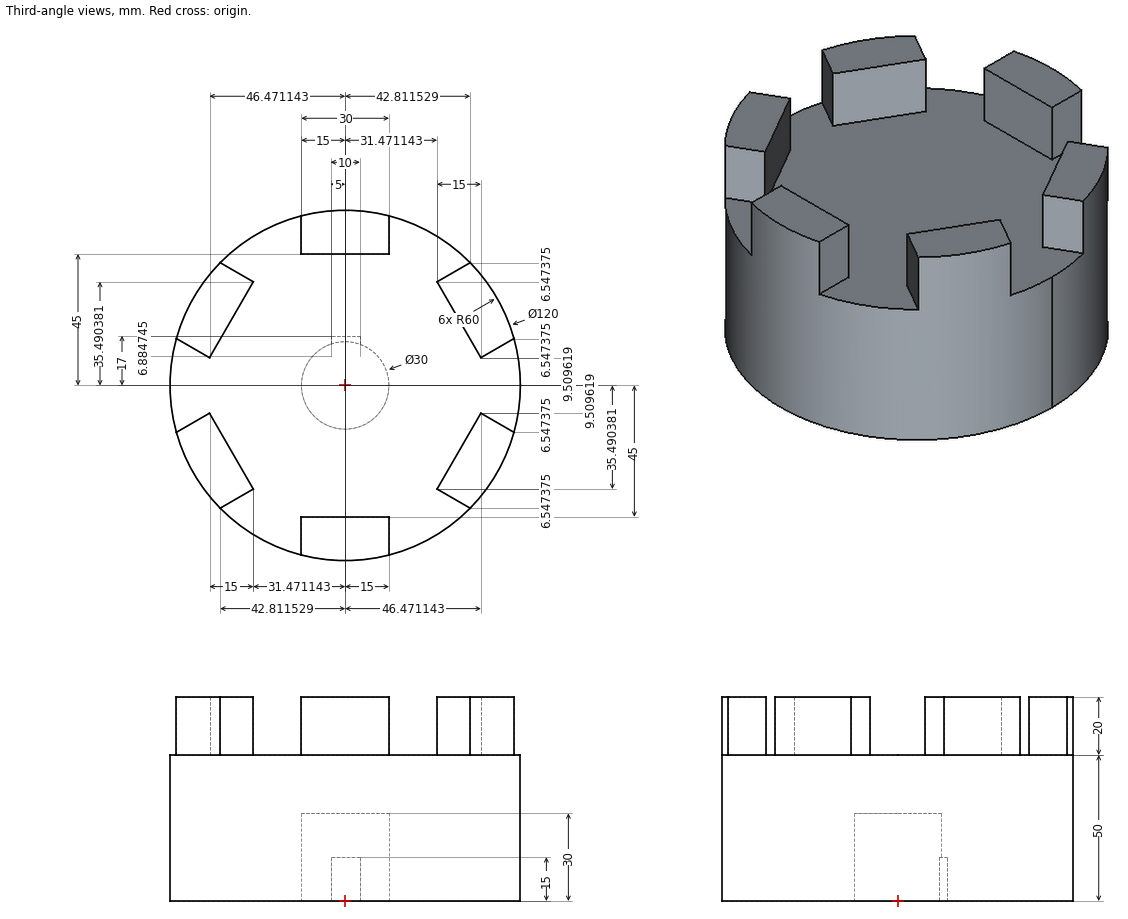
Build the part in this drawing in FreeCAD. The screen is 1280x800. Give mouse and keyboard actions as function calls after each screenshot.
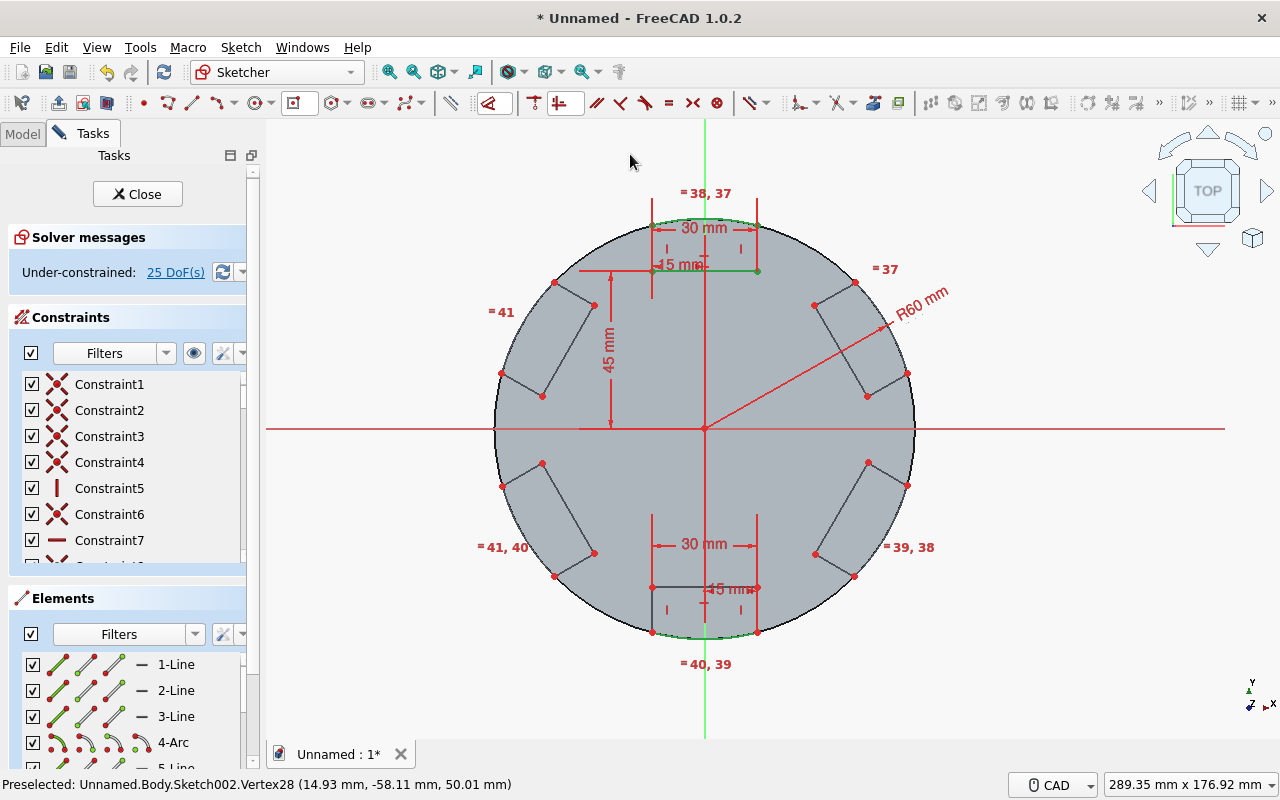
click(757, 587)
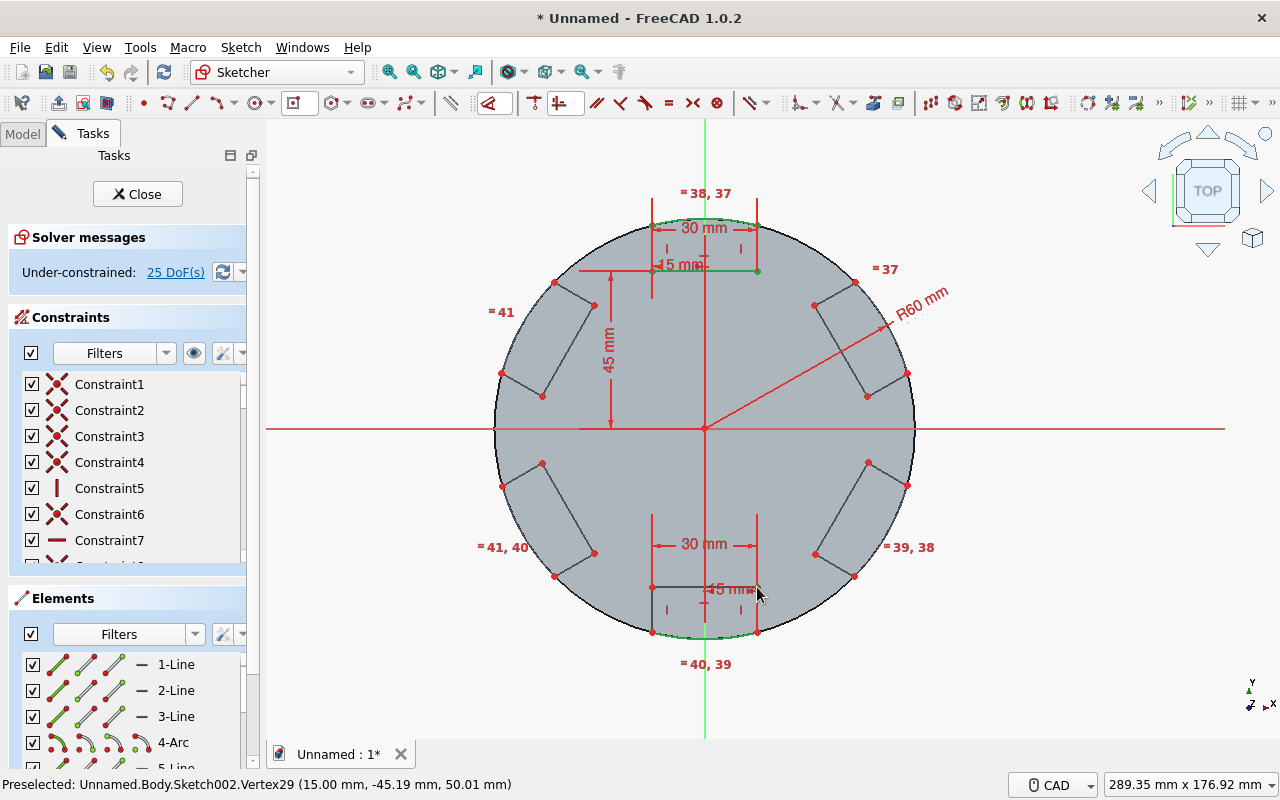
key(i)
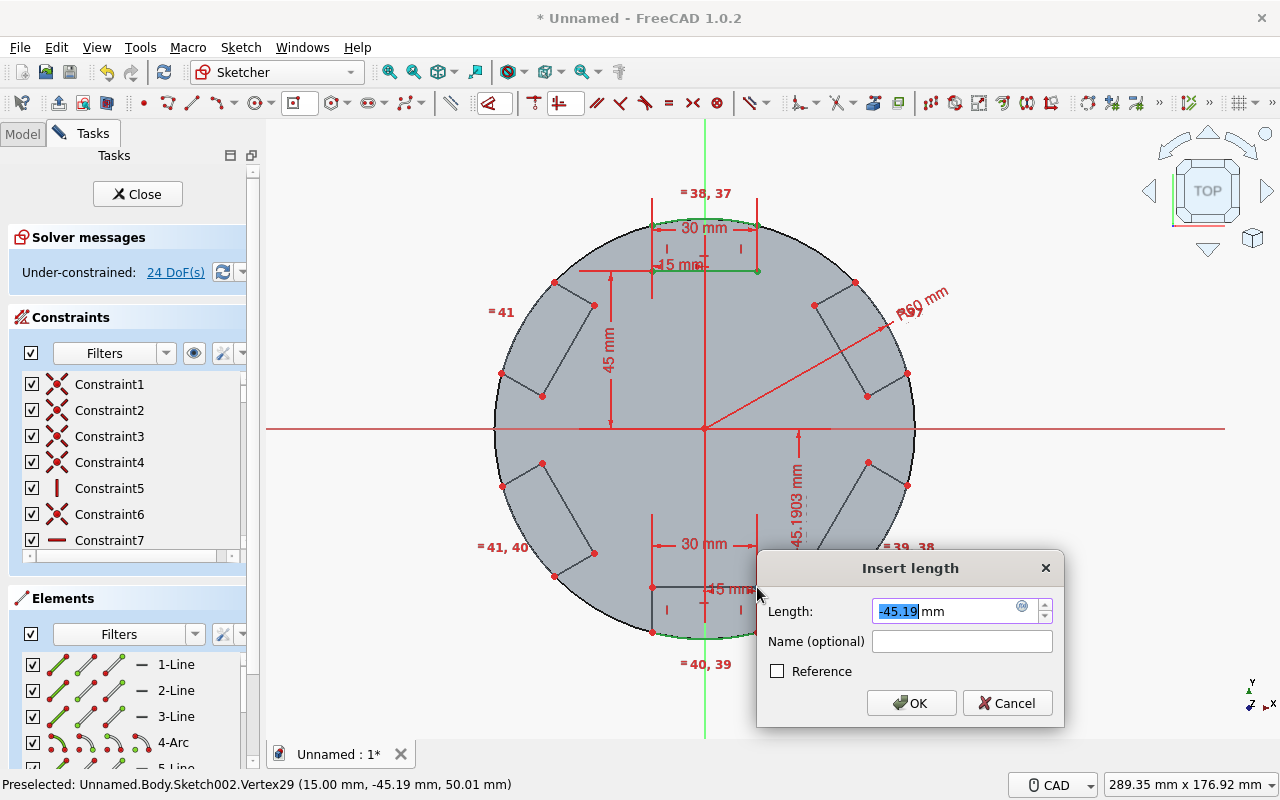
text(-45)
key(Return)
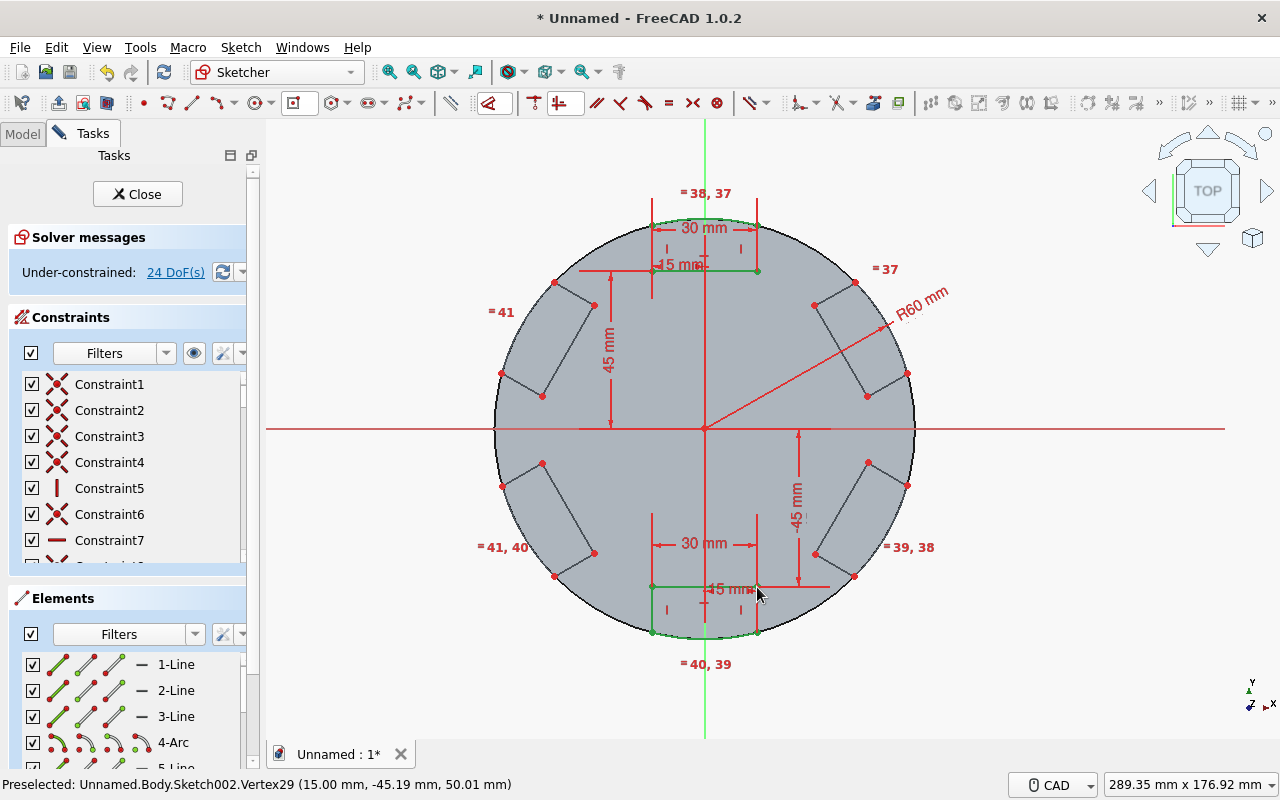
click(831, 333)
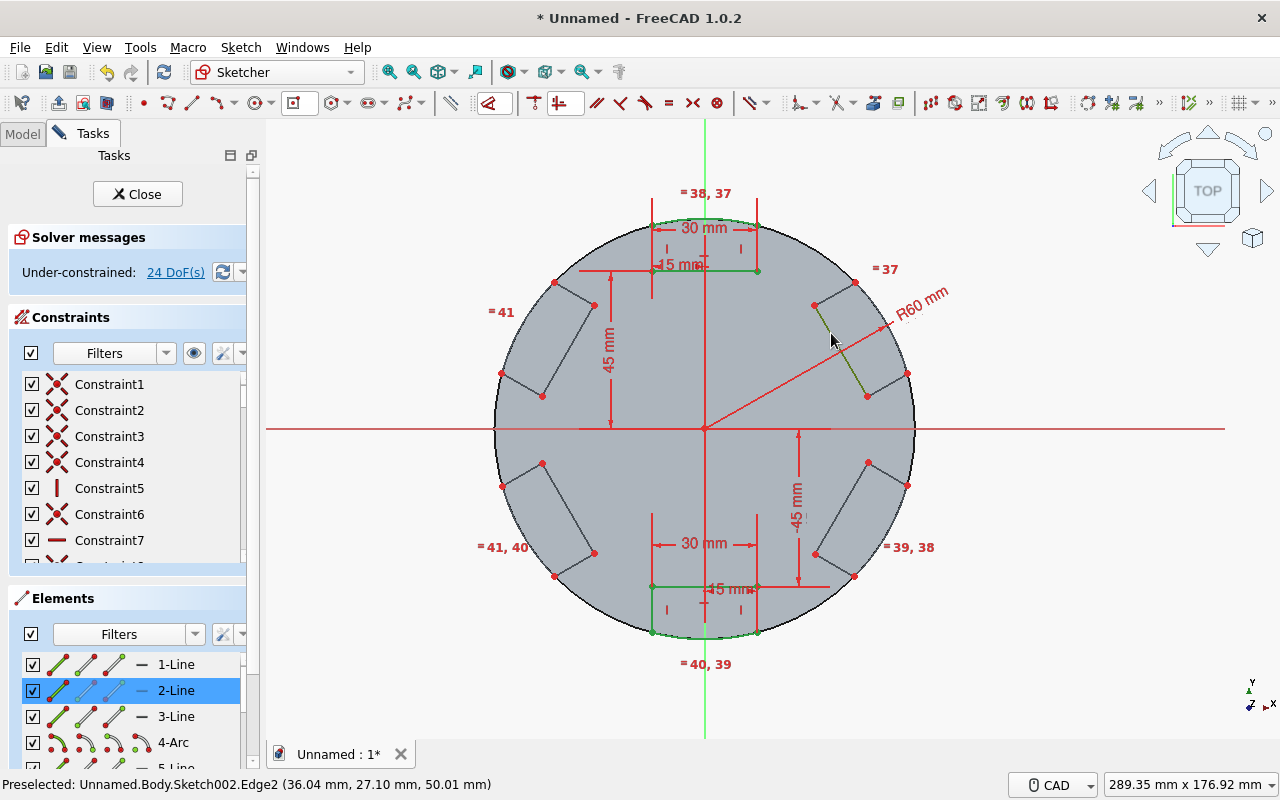
key(l)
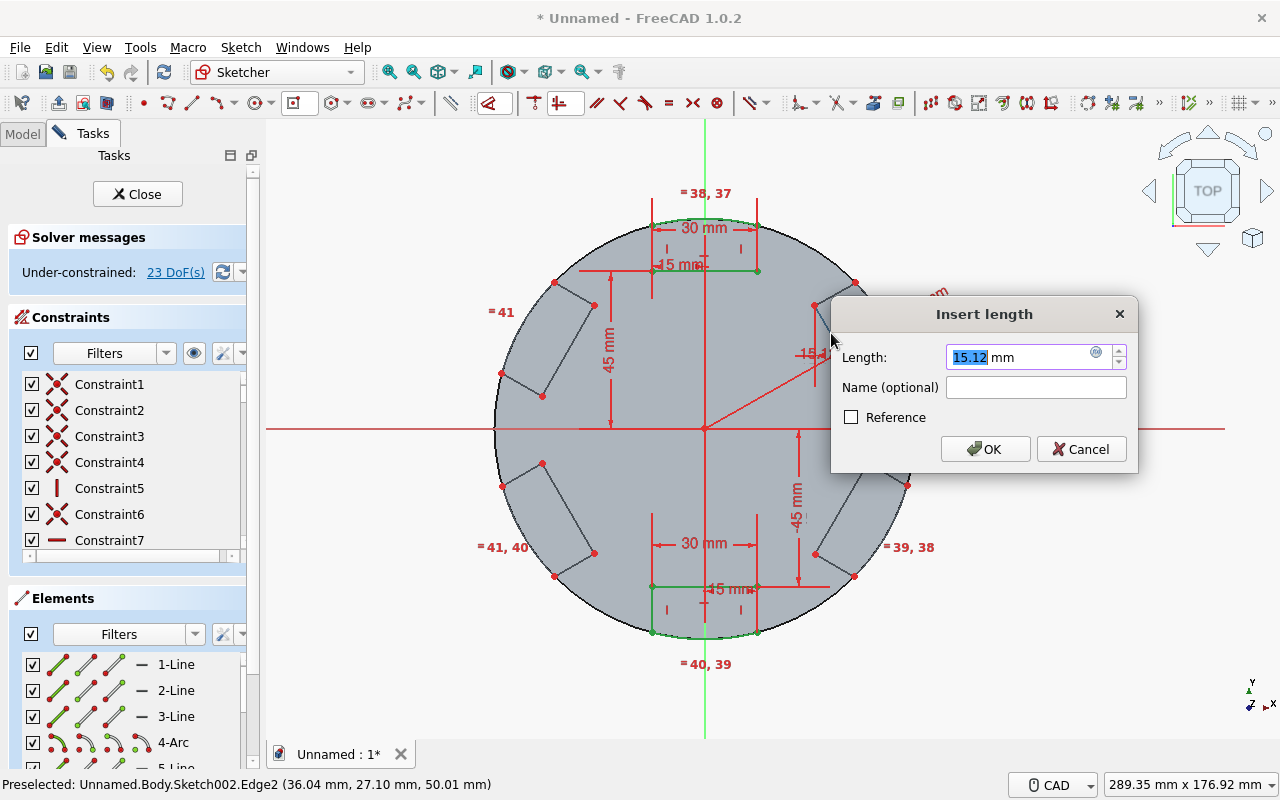
text(15)
key(Return)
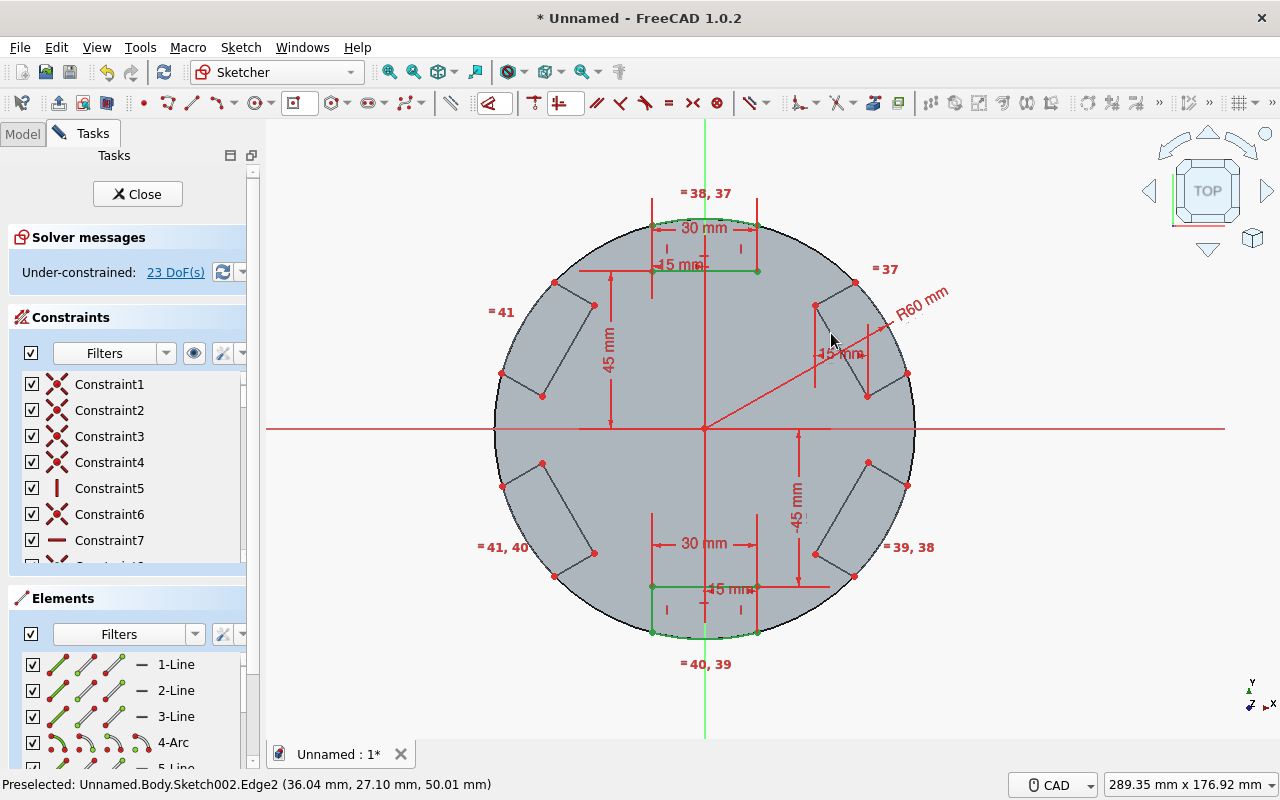
click(852, 490)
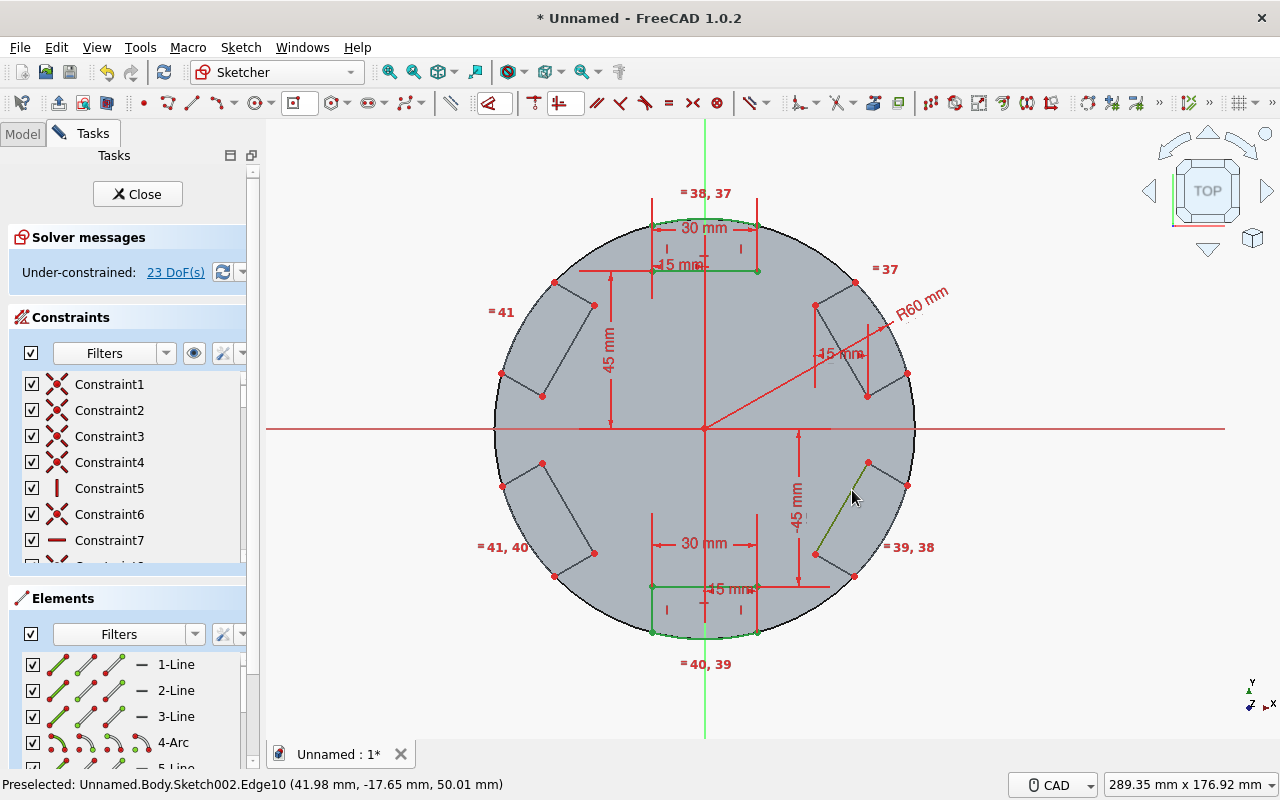
key(l)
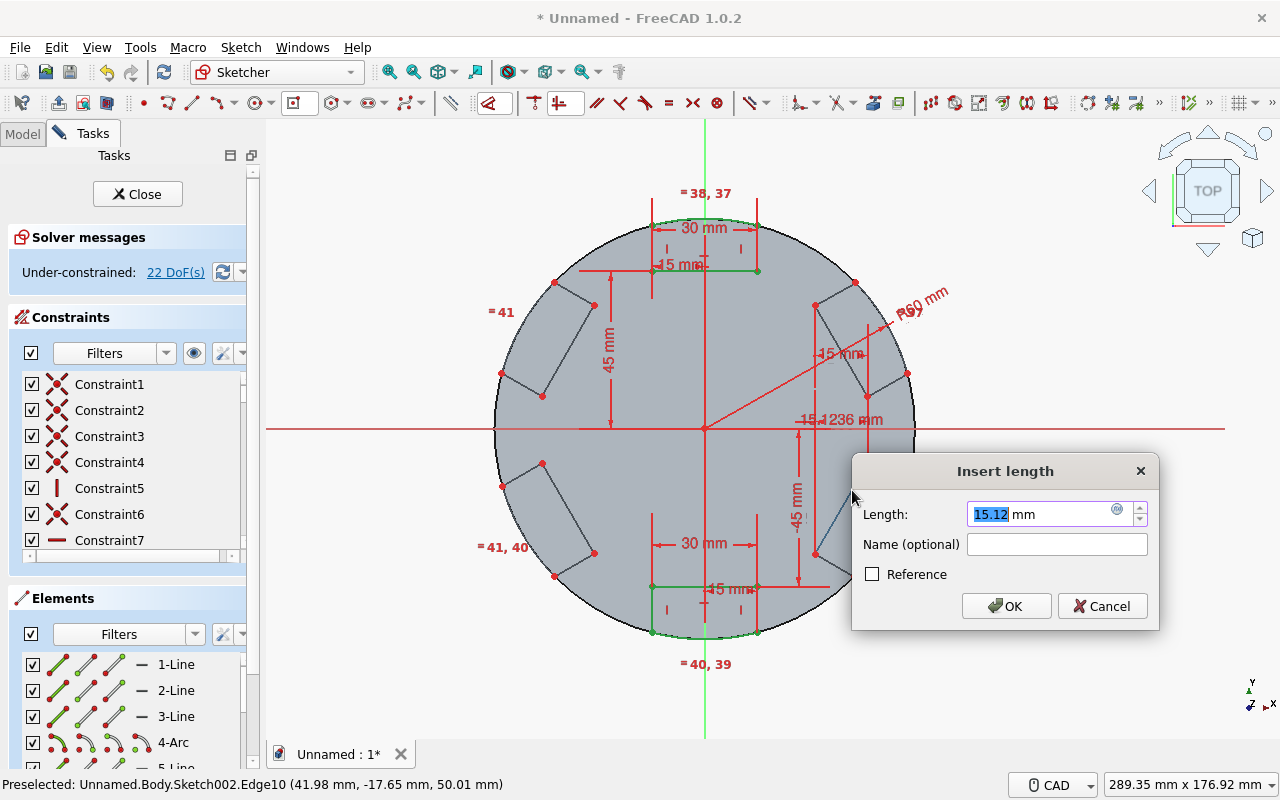
text(15)
key(Return)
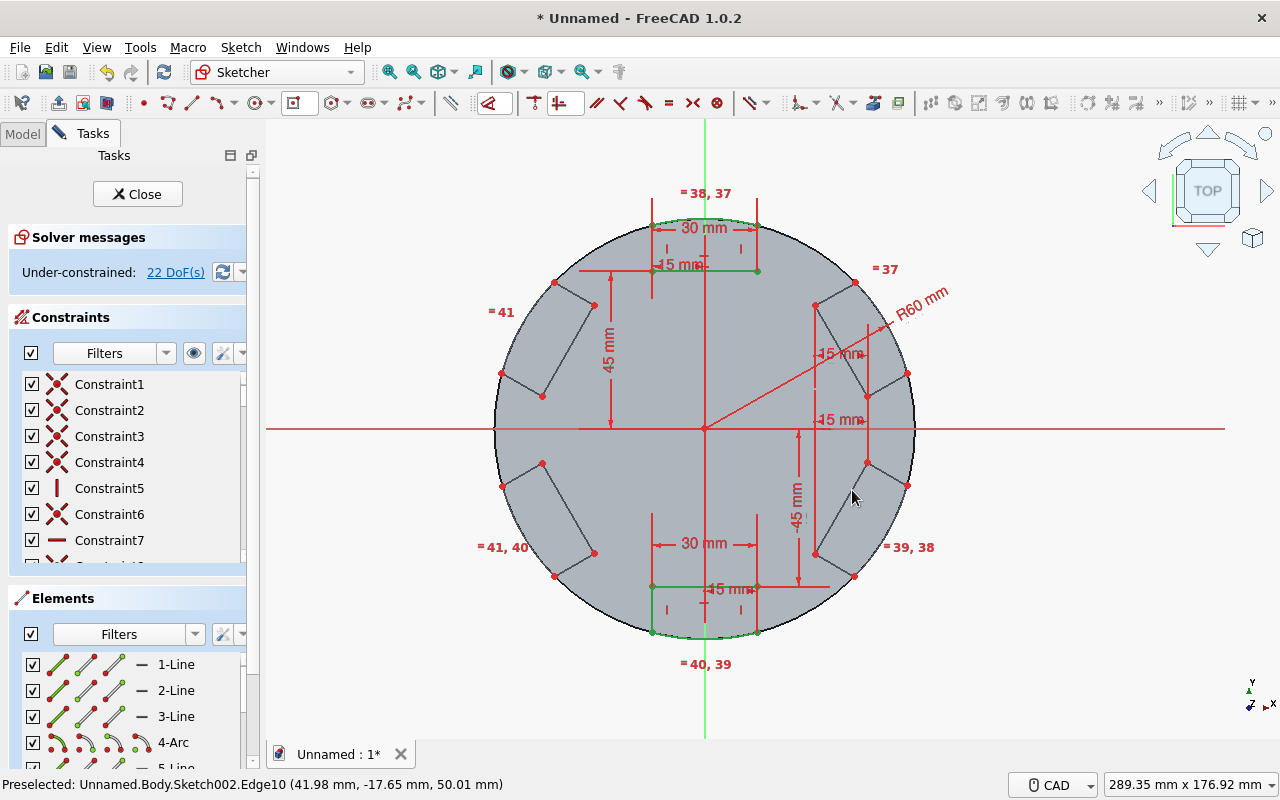
click(579, 527)